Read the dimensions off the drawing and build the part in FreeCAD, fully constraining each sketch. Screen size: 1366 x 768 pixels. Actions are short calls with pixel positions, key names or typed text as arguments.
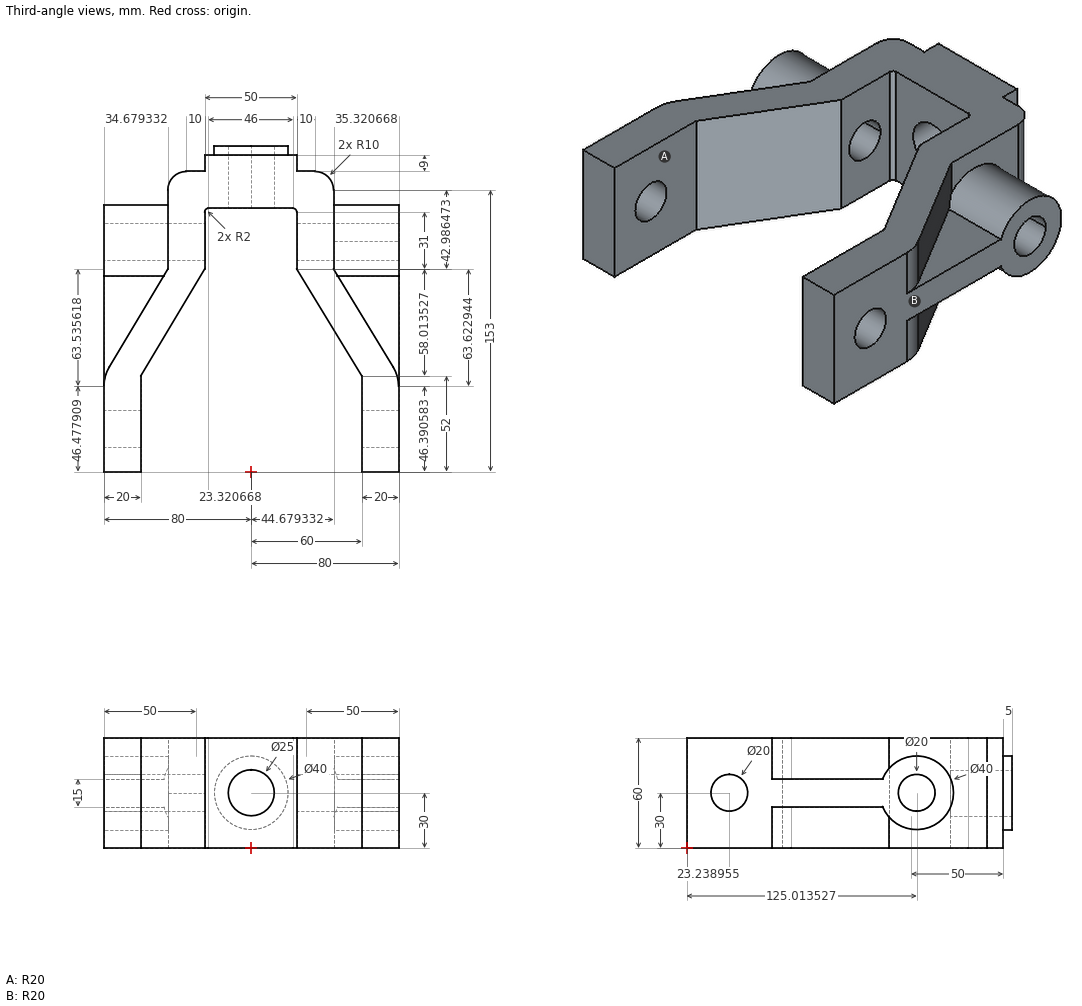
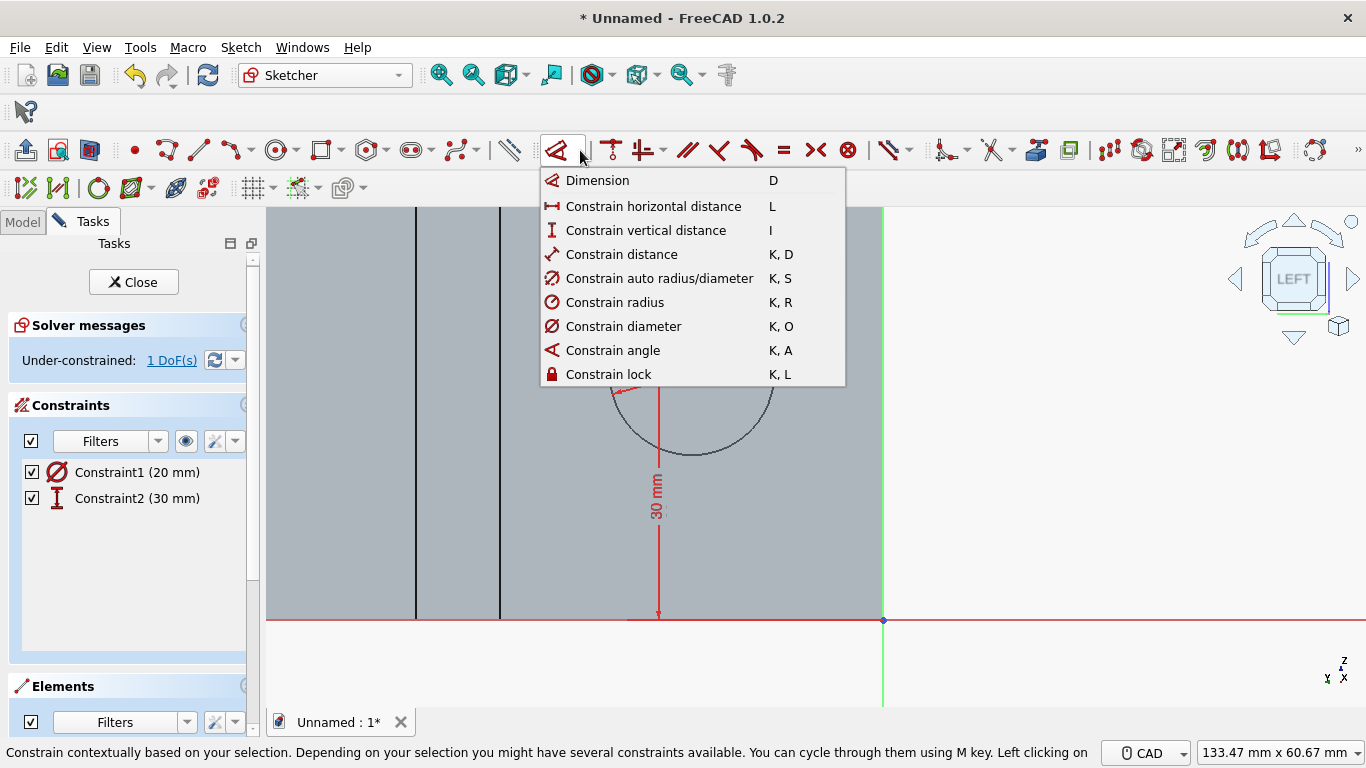
click(693, 206)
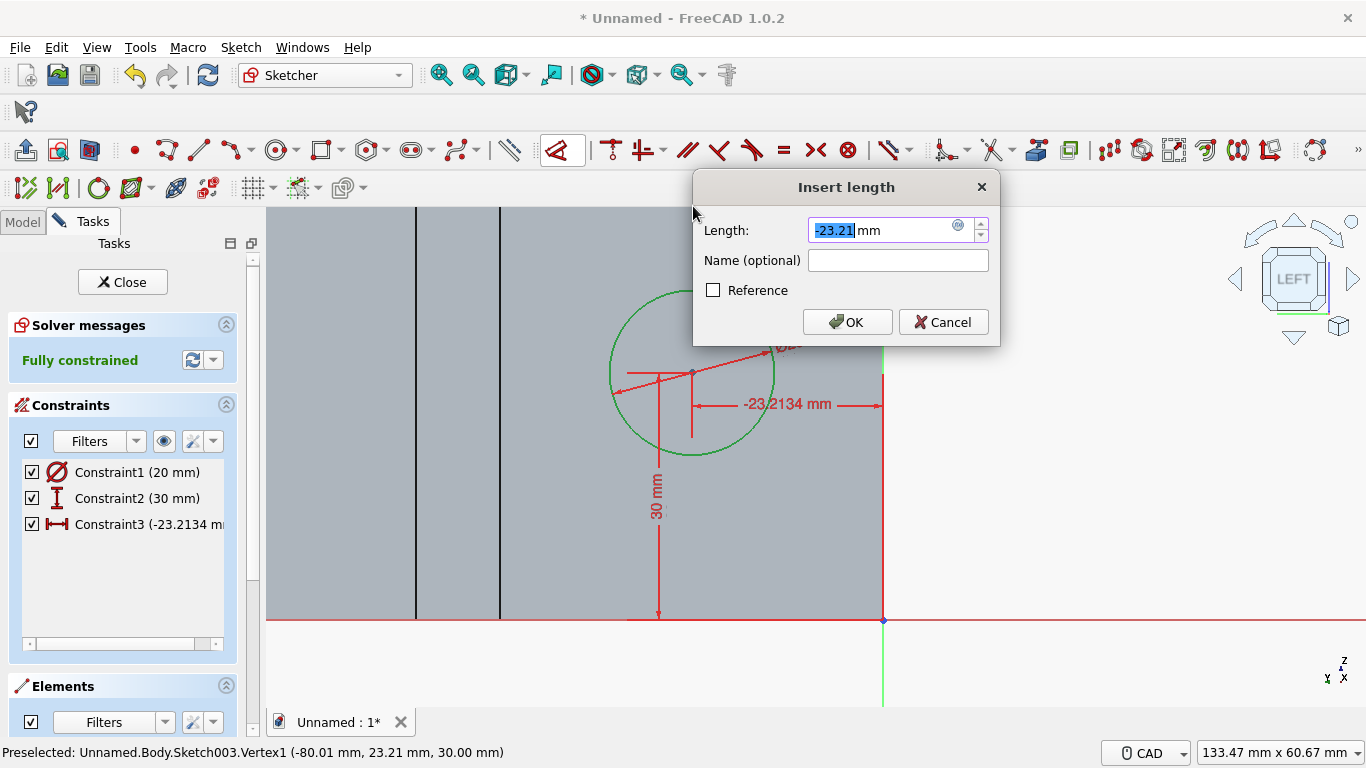
text(-23.238955)
key(Return)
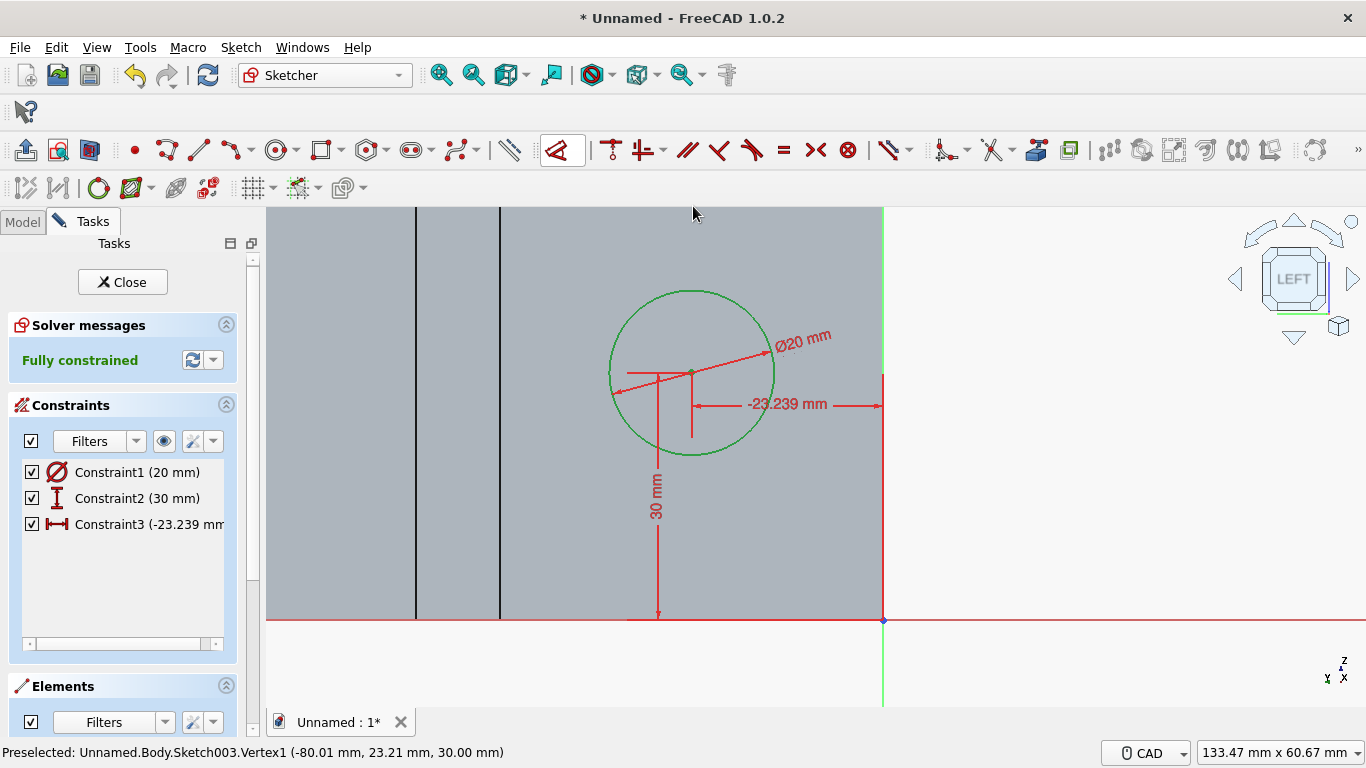
click(123, 282)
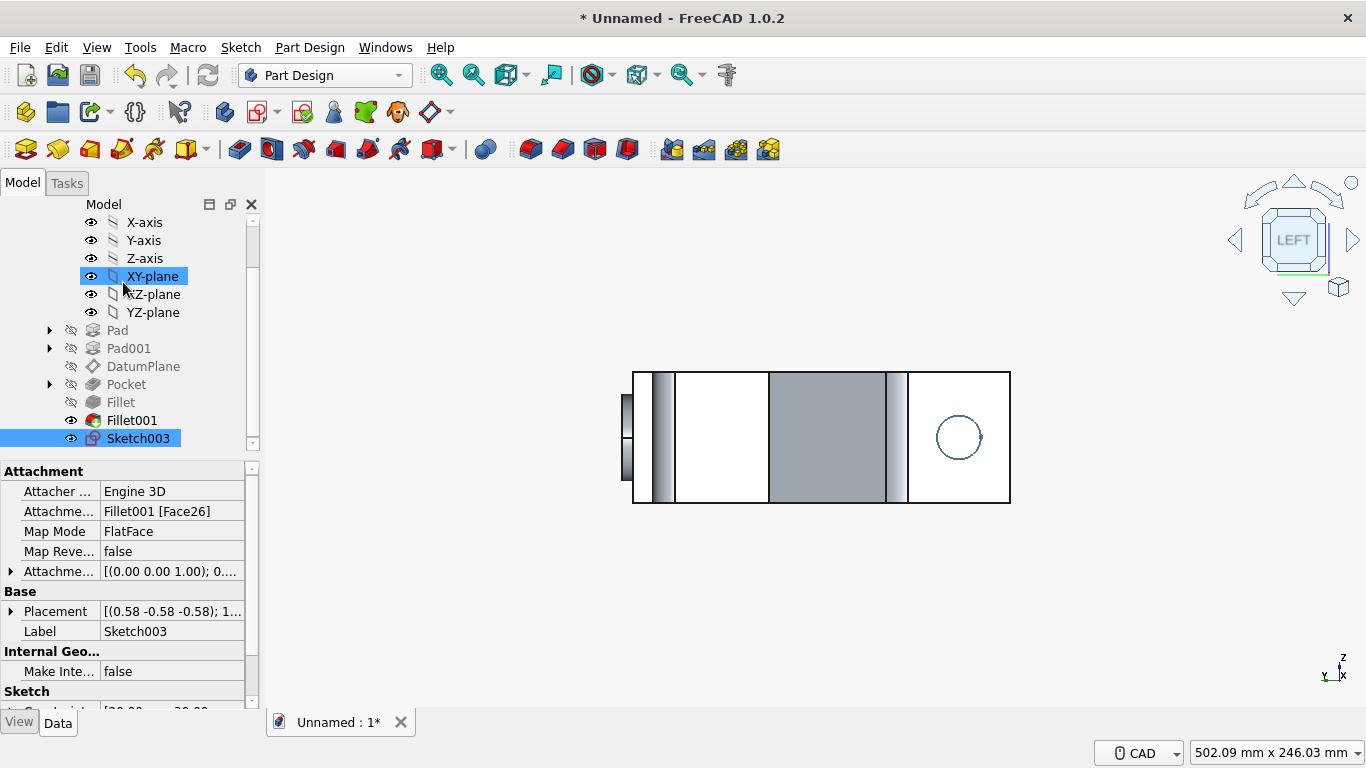
click(240, 150)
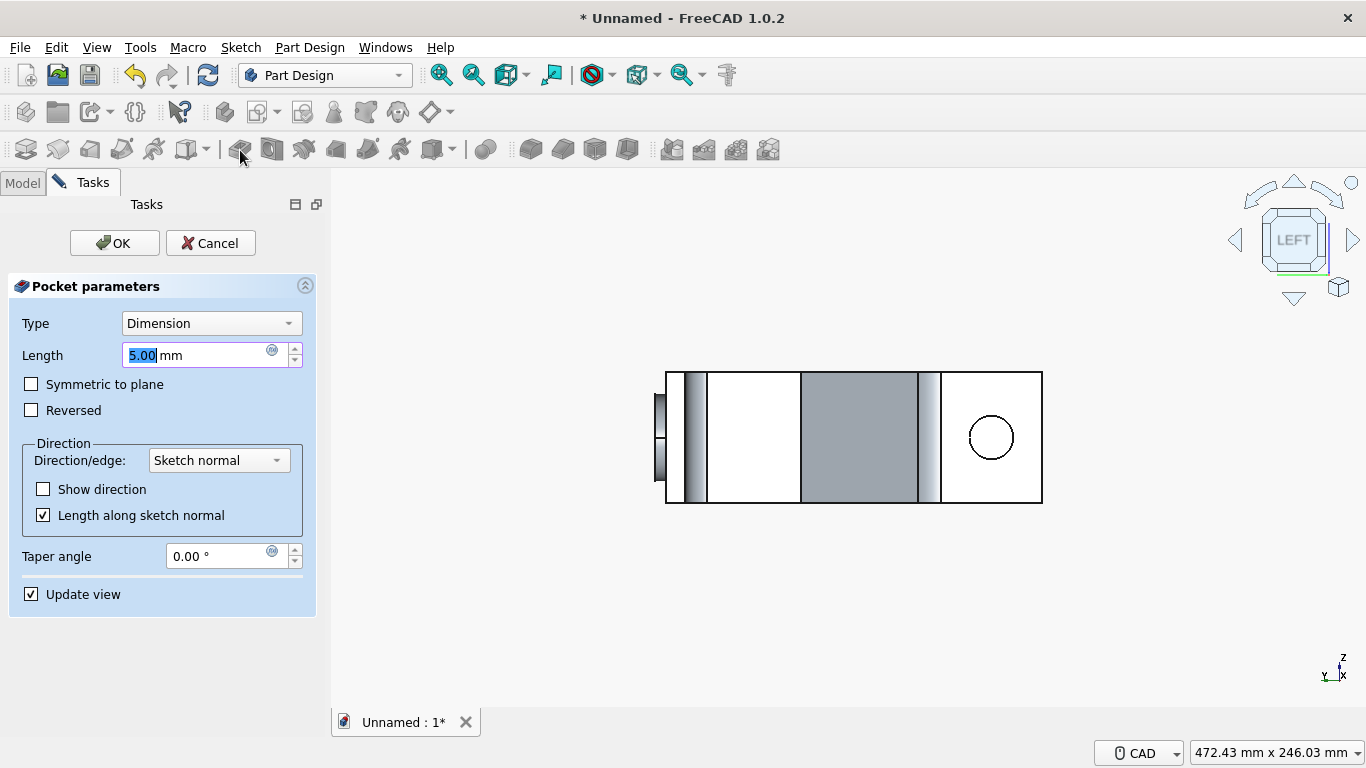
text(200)
key(Tab)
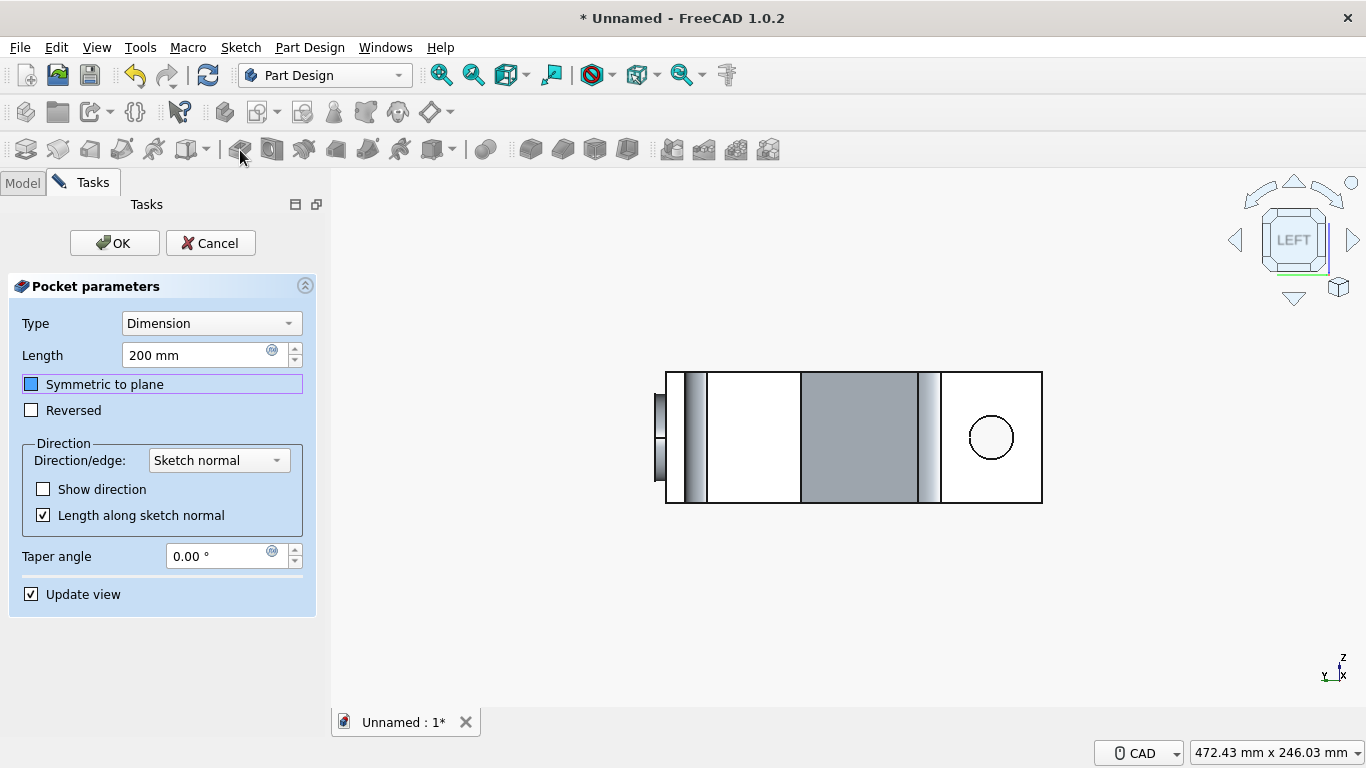
click(115, 243)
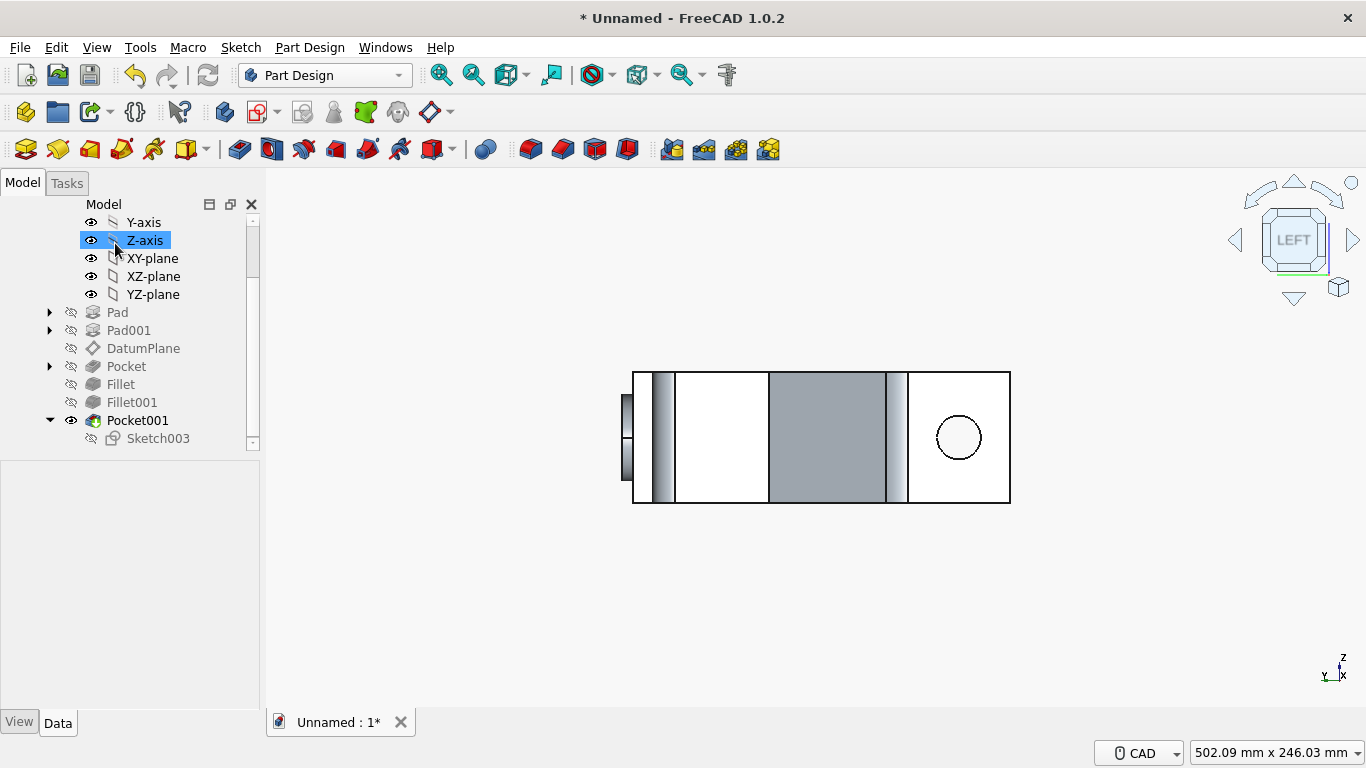
key(v)
key(f)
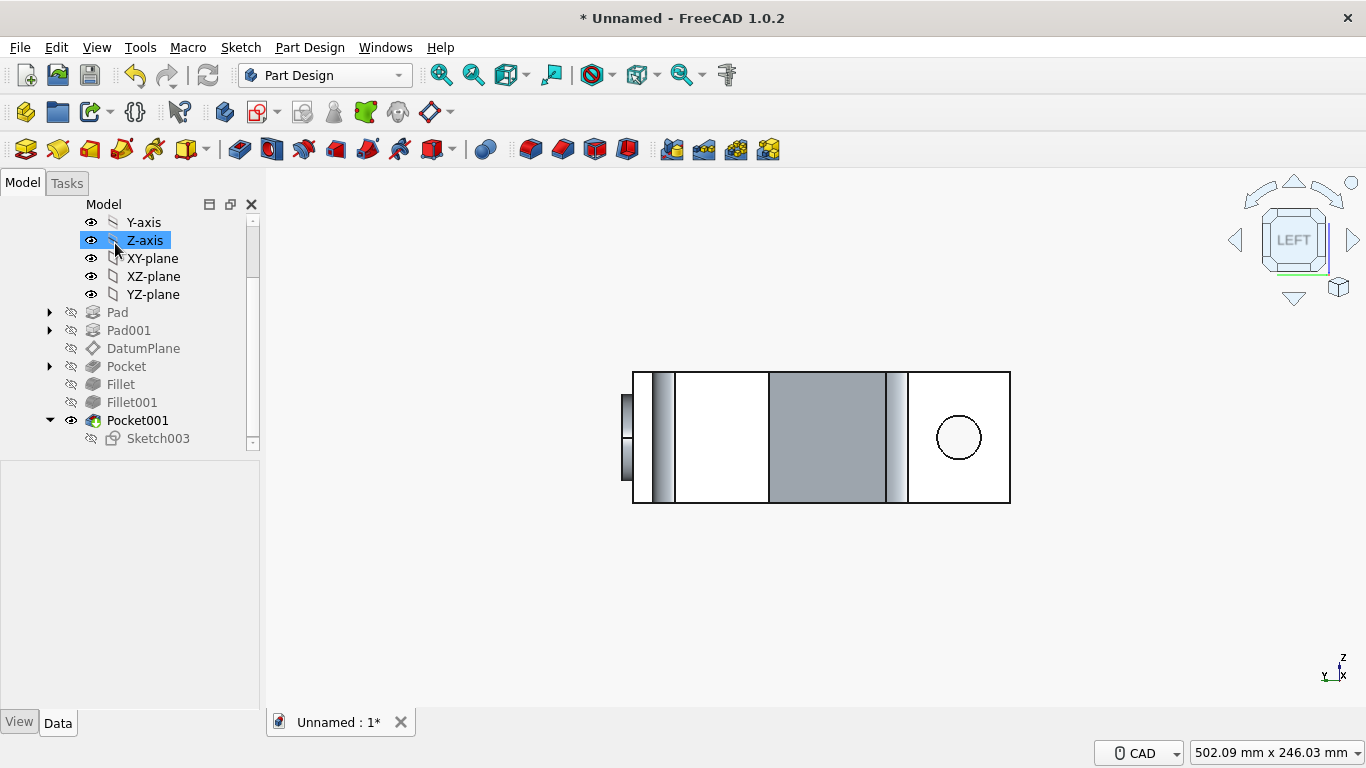
scroll(160, 326, down, 3)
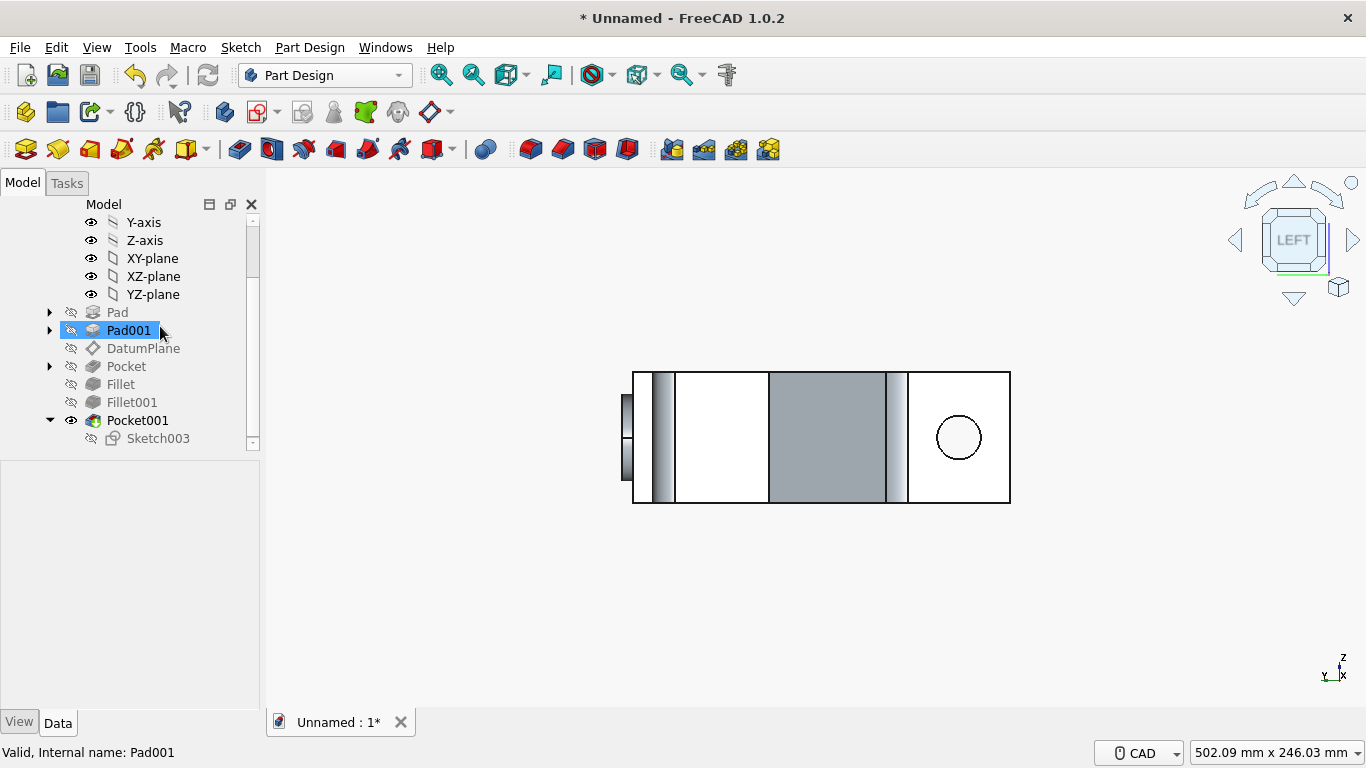
scroll(160, 326, up, 15)